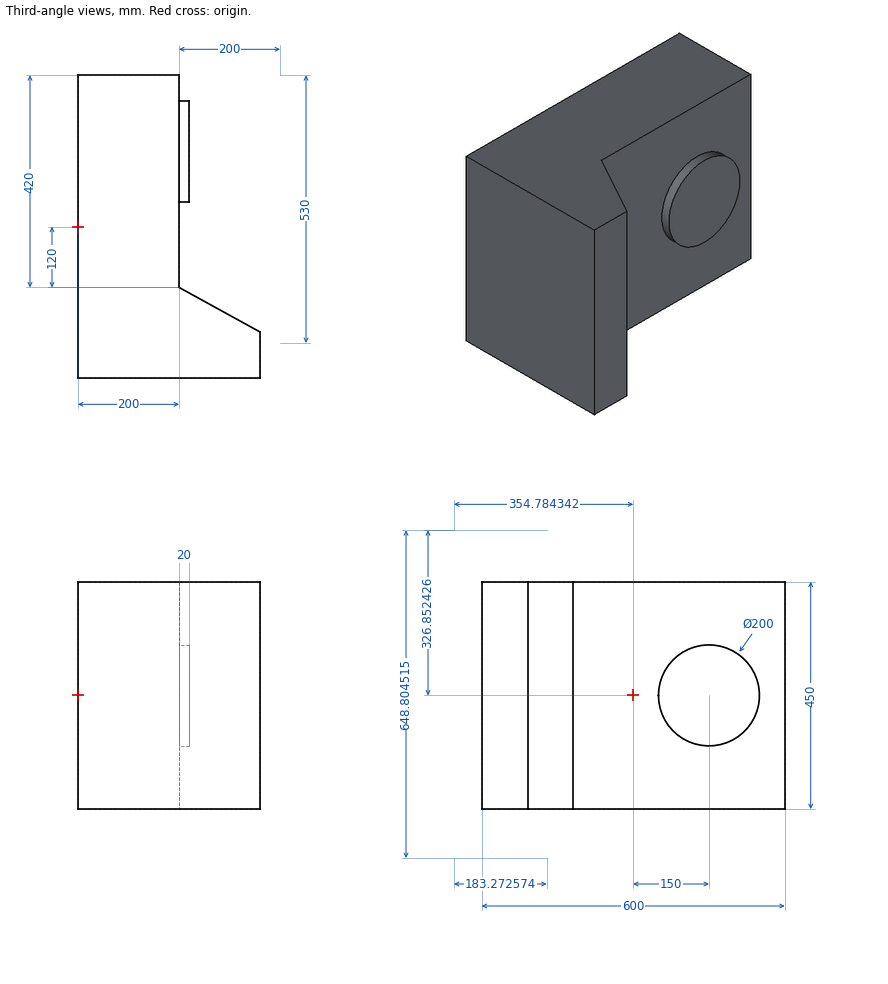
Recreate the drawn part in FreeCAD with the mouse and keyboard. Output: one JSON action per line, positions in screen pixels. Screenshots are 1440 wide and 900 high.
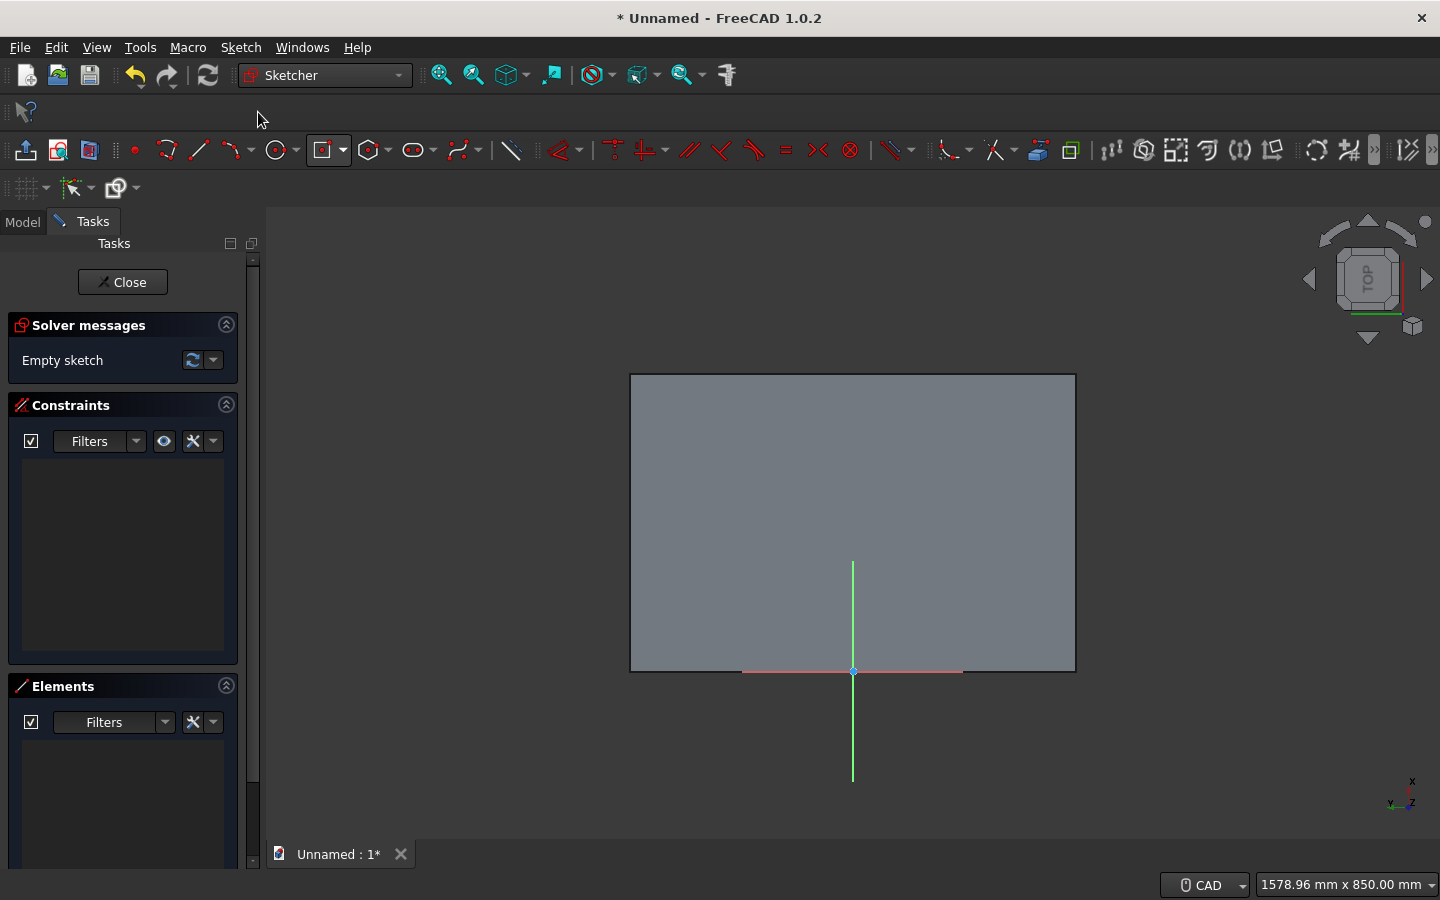
{"action": "scroll", "coordinate": [913, 523], "scroll_direction": "up", "scroll_amount": 2}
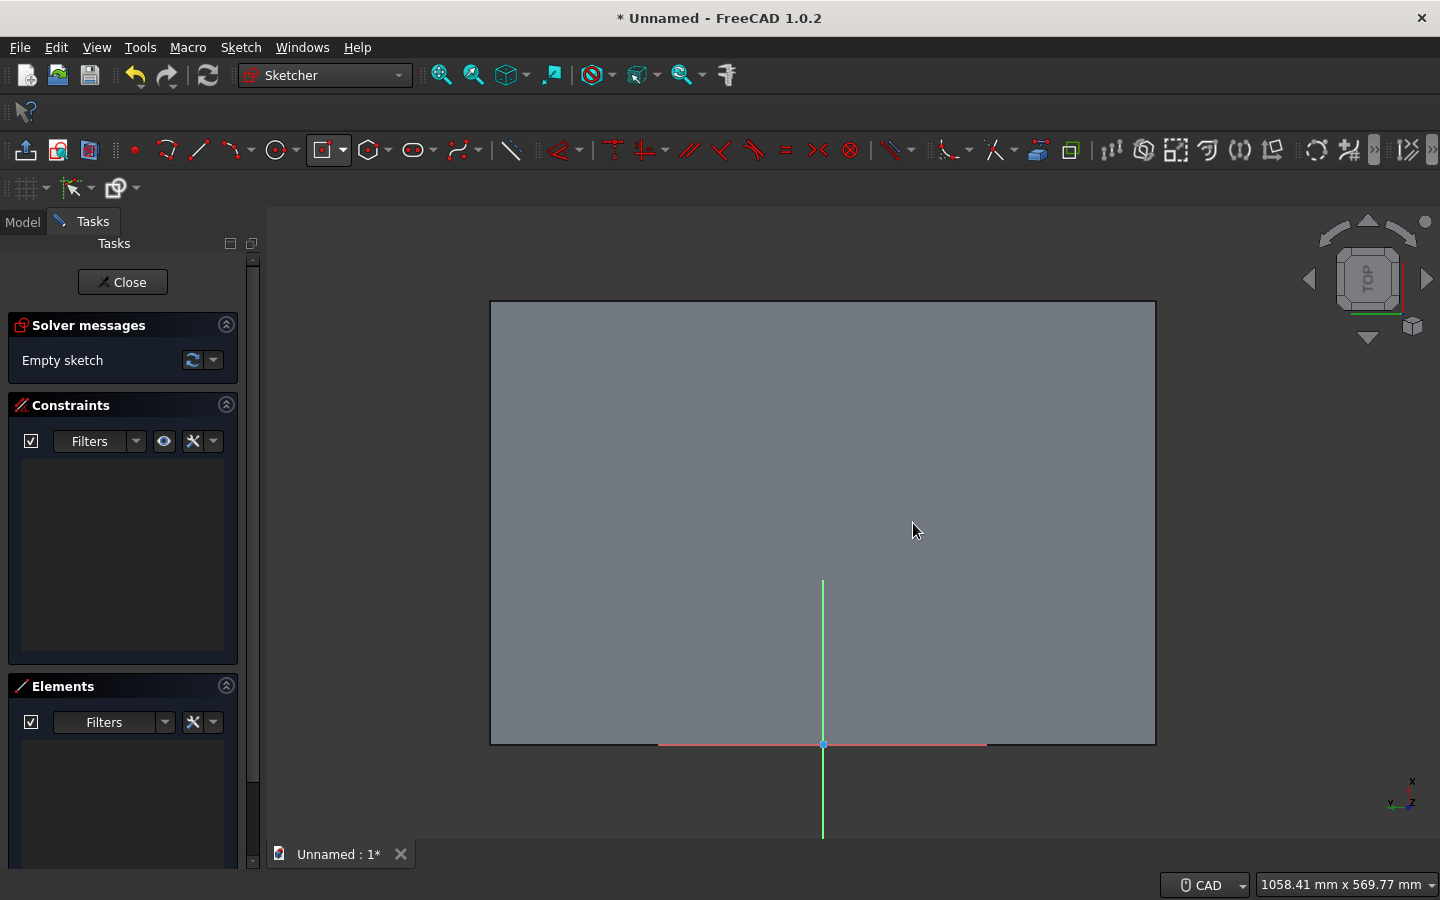
{"action": "key", "text": "g m"}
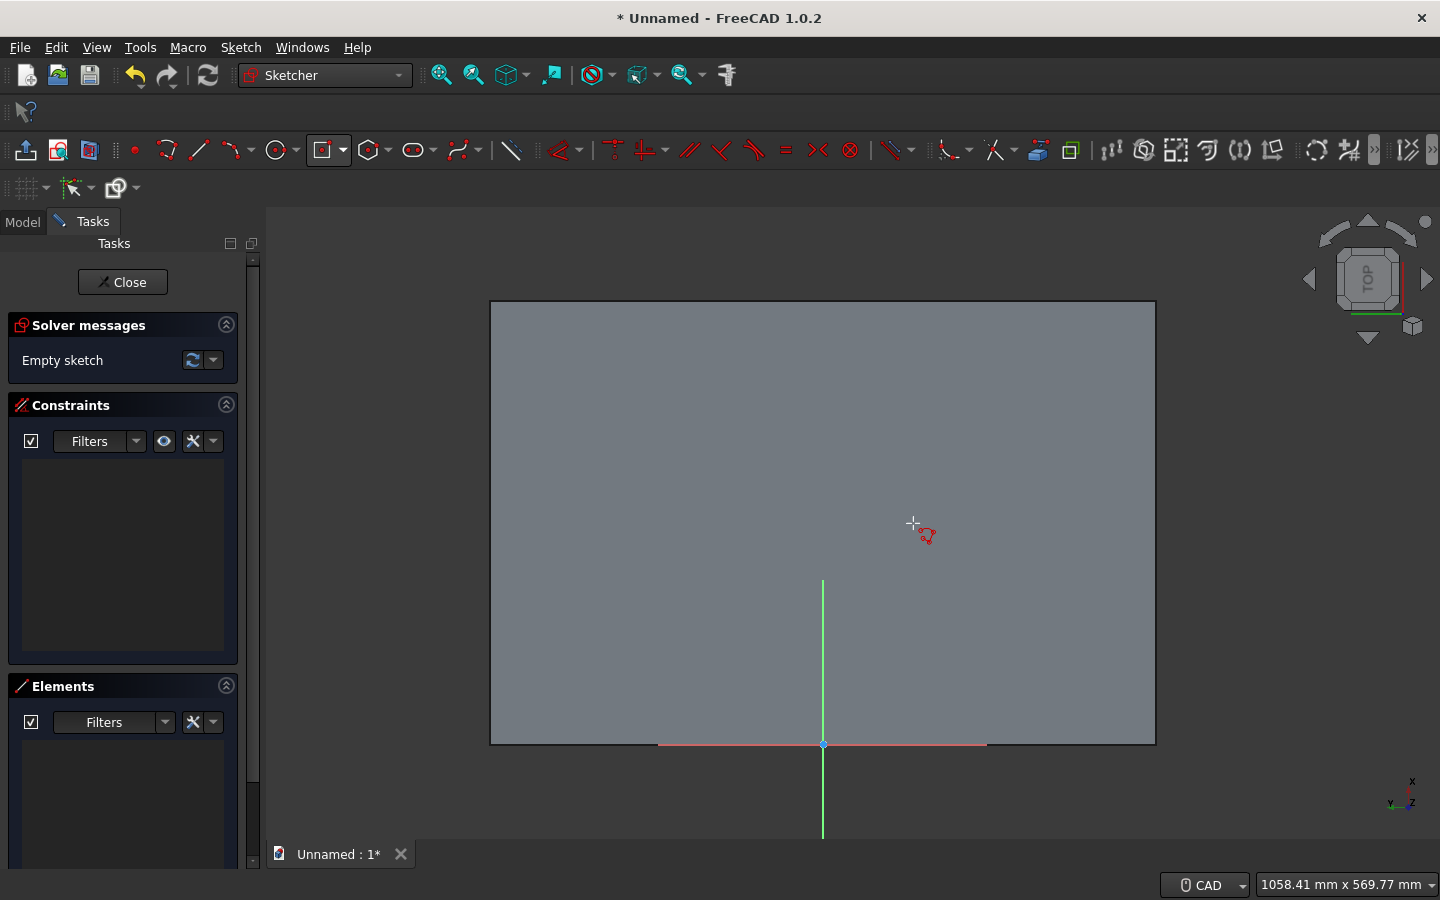
{"action": "left_click", "coordinate": [956, 523]}
{"action": "left_click", "coordinate": [1078, 301]}
{"action": "left_click", "coordinate": [490, 301]}
{"action": "left_click", "coordinate": [490, 523]}
{"action": "left_click", "coordinate": [956, 524]}
{"action": "key", "text": "Escape"}
{"action": "key", "text": "Escape"}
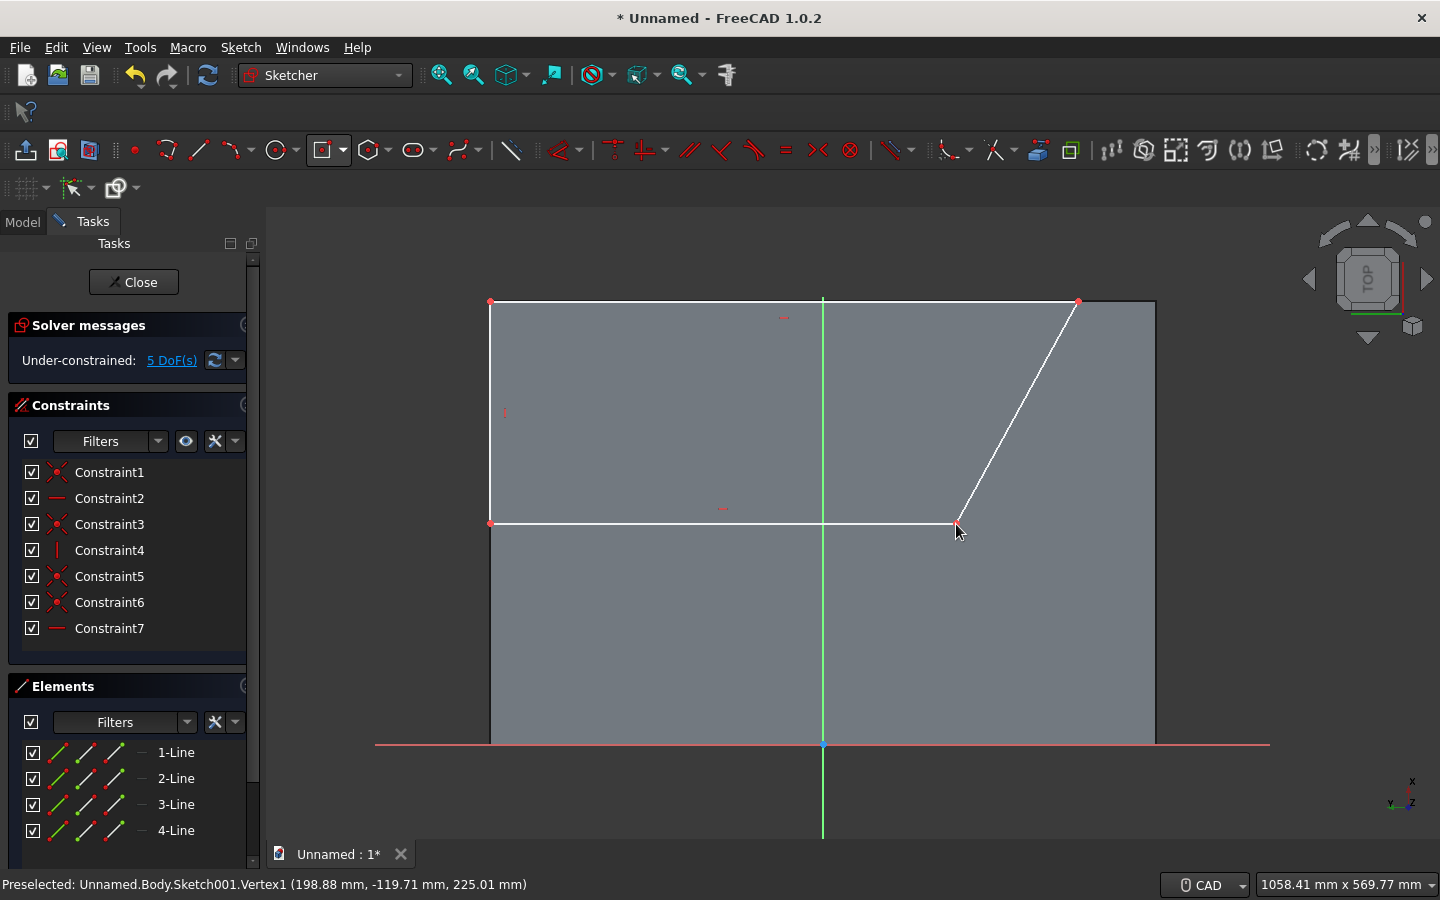
{"action": "key", "text": "d"}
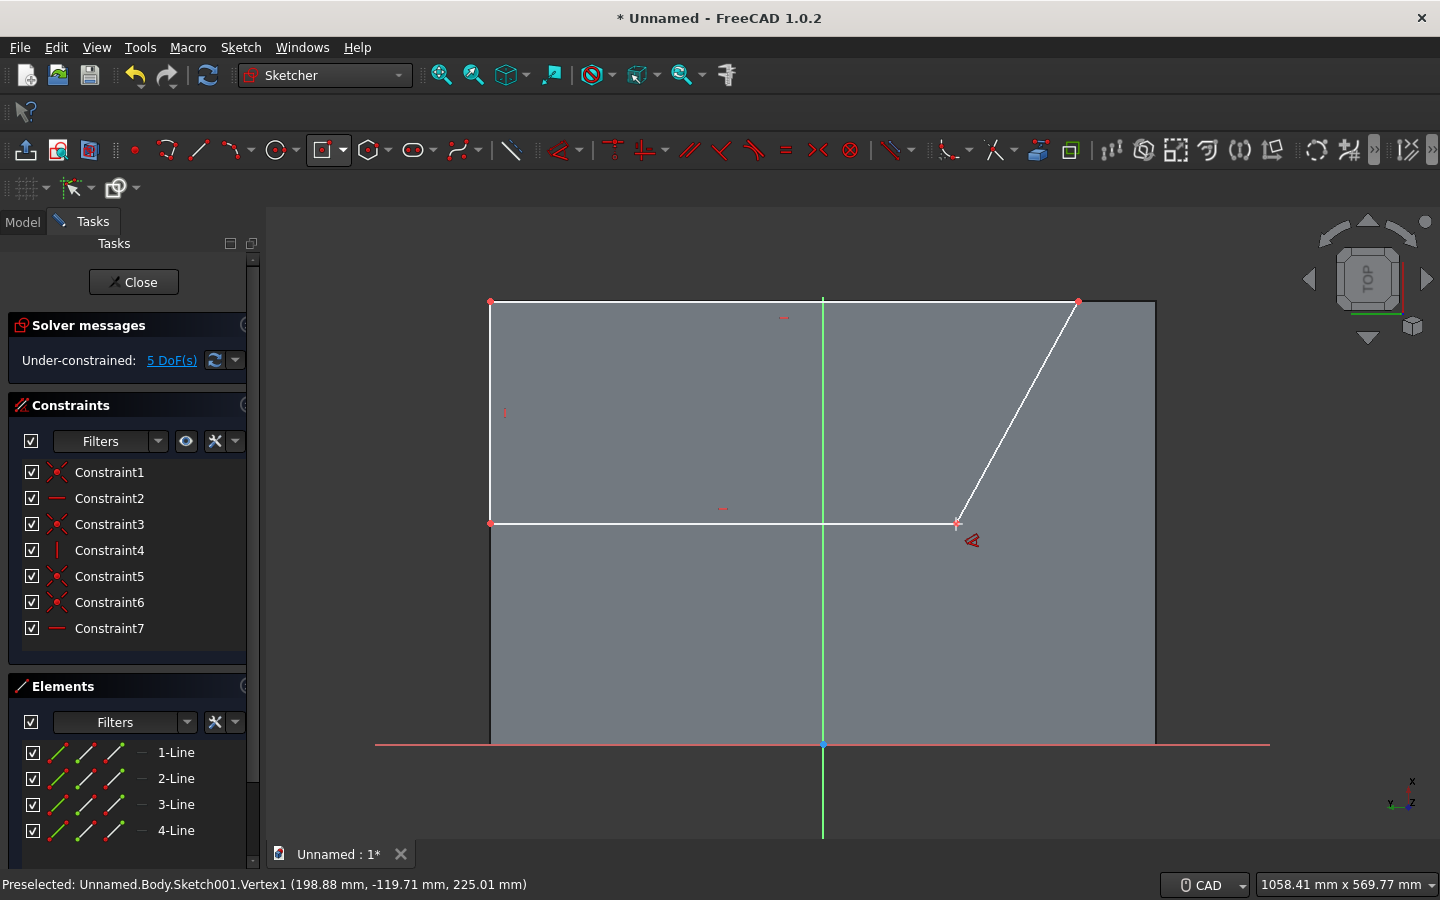
{"action": "left_click", "coordinate": [902, 302]}
{"action": "left_click", "coordinate": [784, 268]}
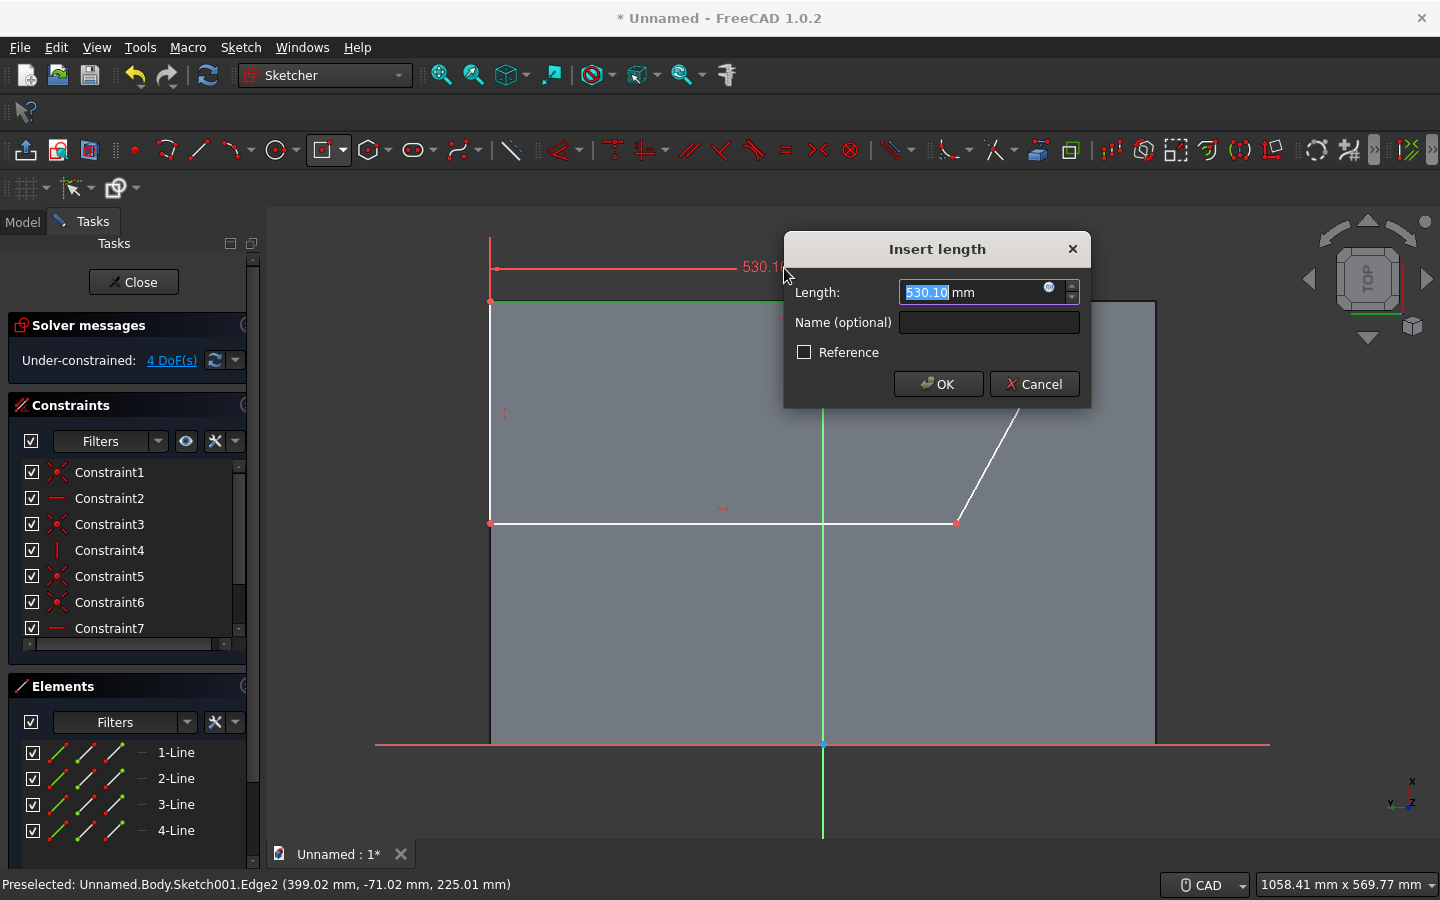
{"action": "type", "text": "530"}
{"action": "key", "text": "Return"}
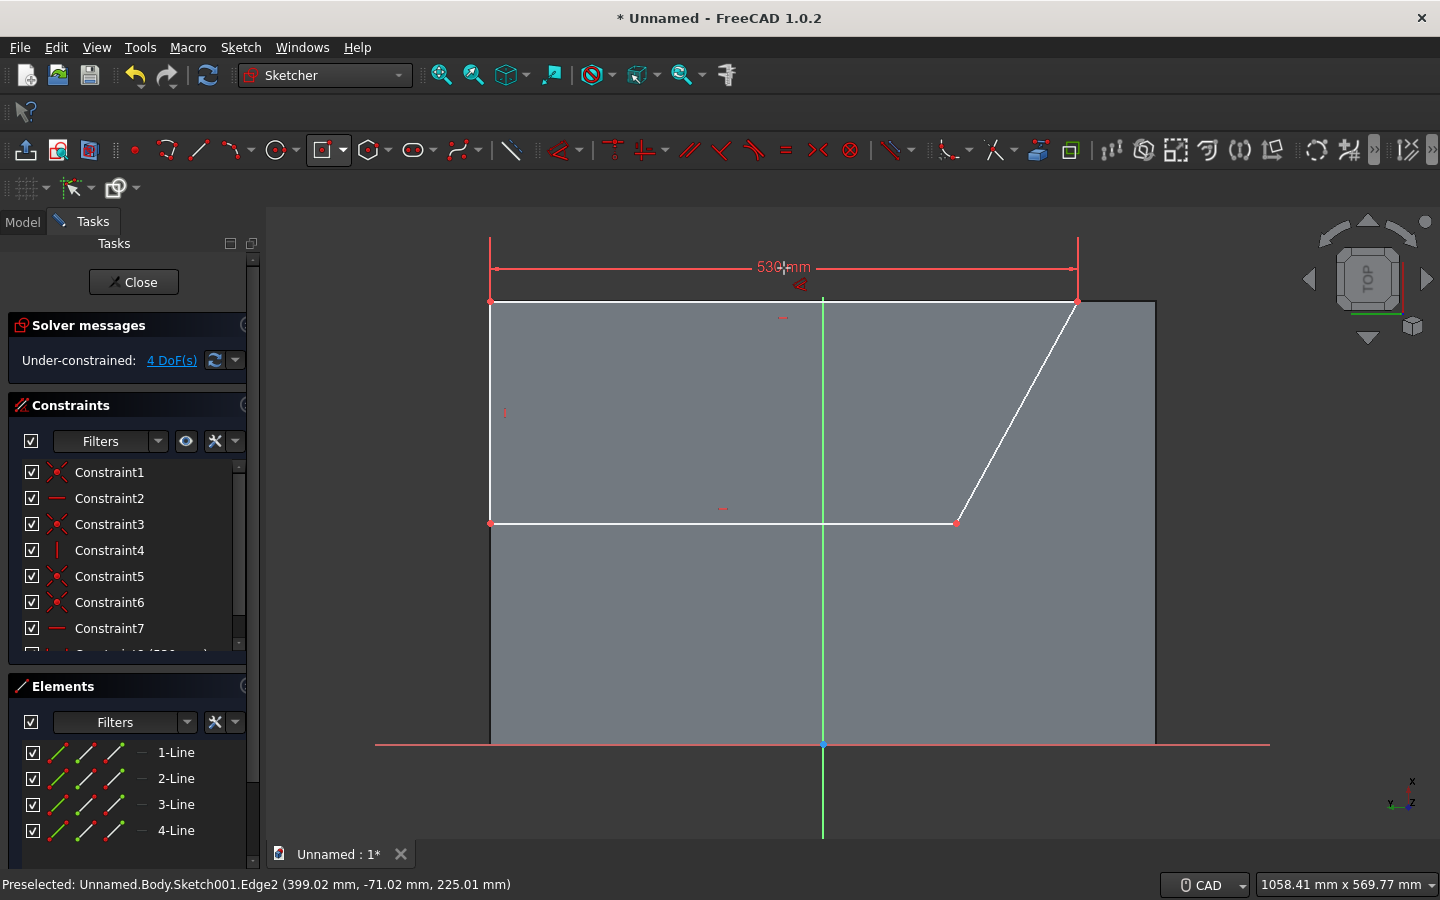
{"action": "left_click", "coordinate": [490, 369]}
{"action": "left_click", "coordinate": [456, 413]}